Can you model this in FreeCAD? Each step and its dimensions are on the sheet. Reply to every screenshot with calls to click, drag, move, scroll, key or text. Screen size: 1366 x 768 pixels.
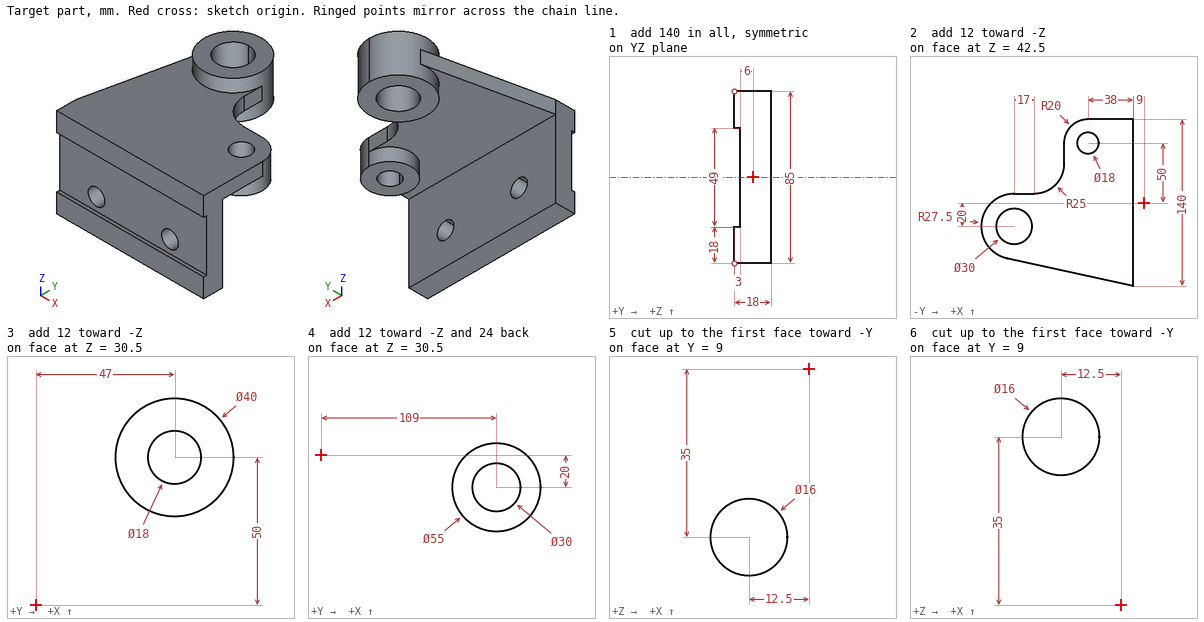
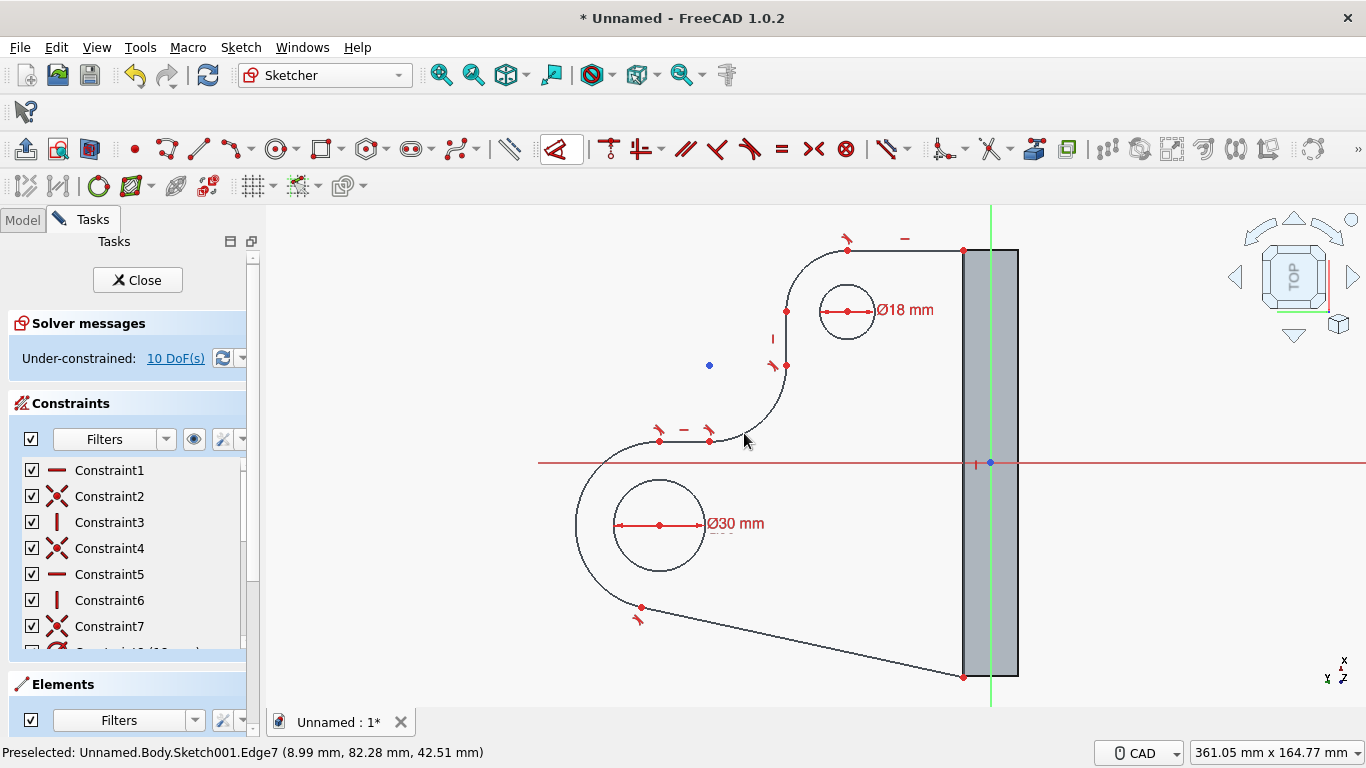
click(786, 349)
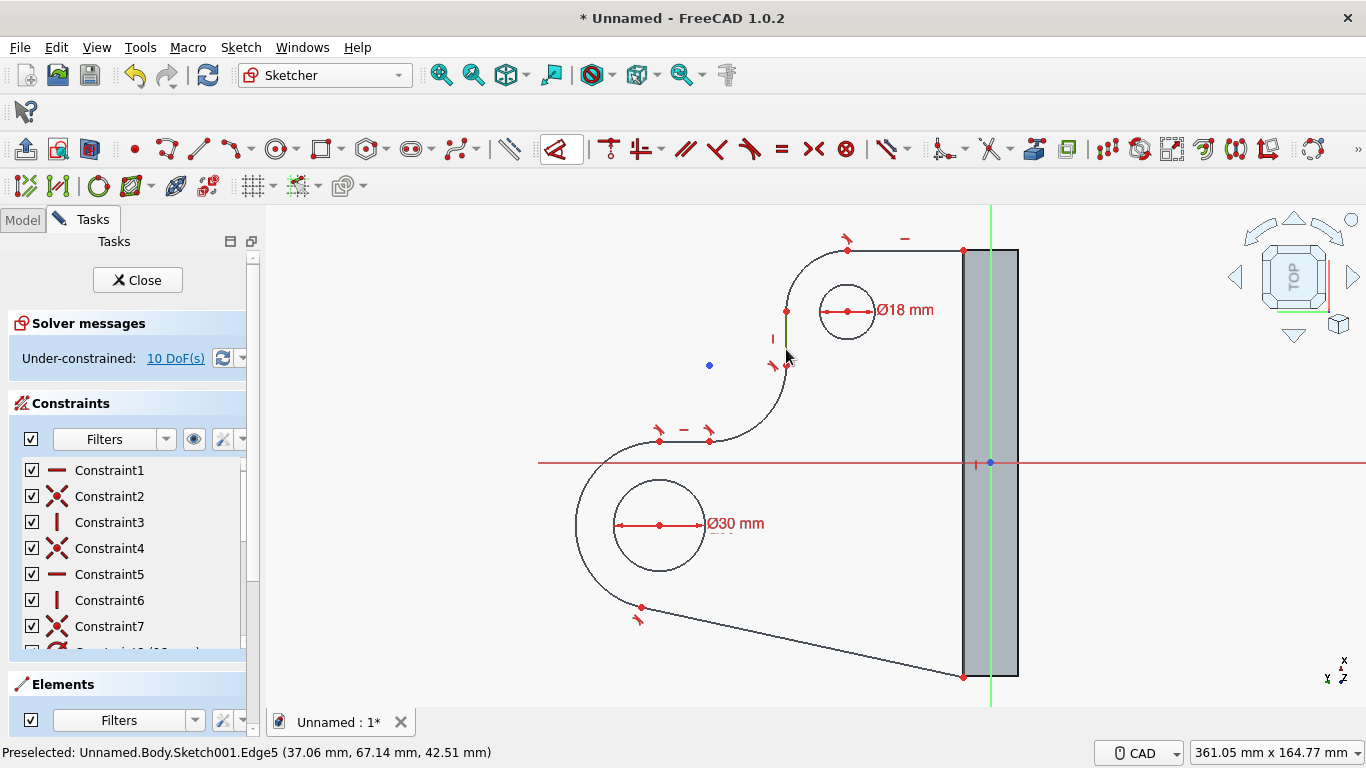
click(820, 257)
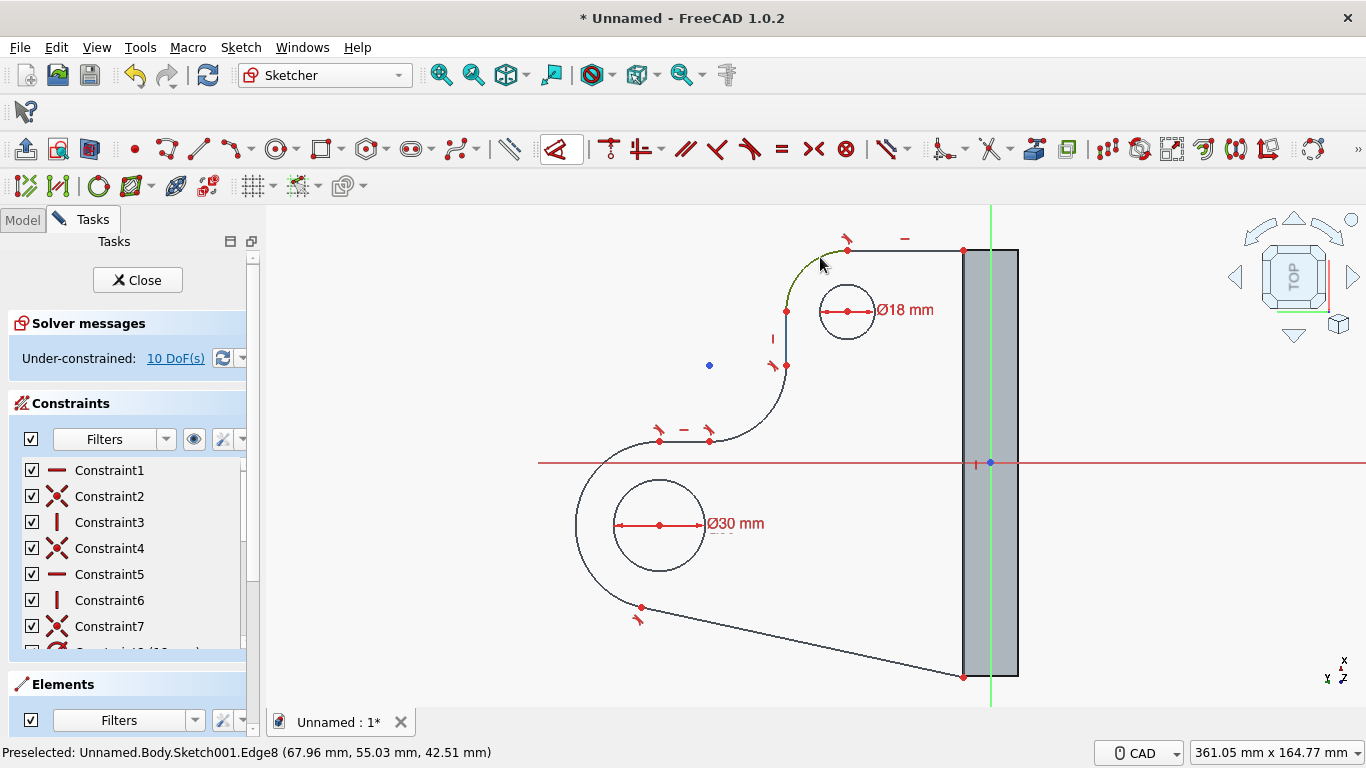
key(t)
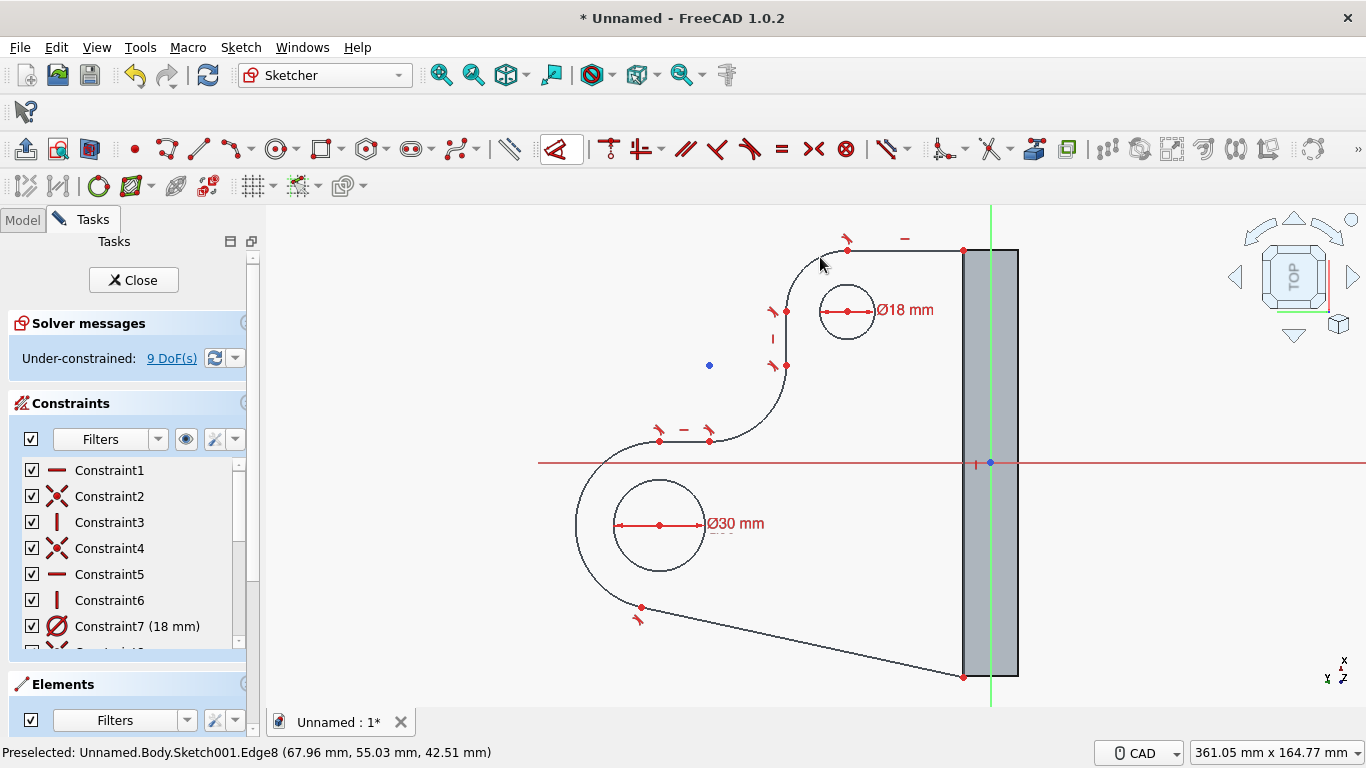
scroll(595, 472, up, 3)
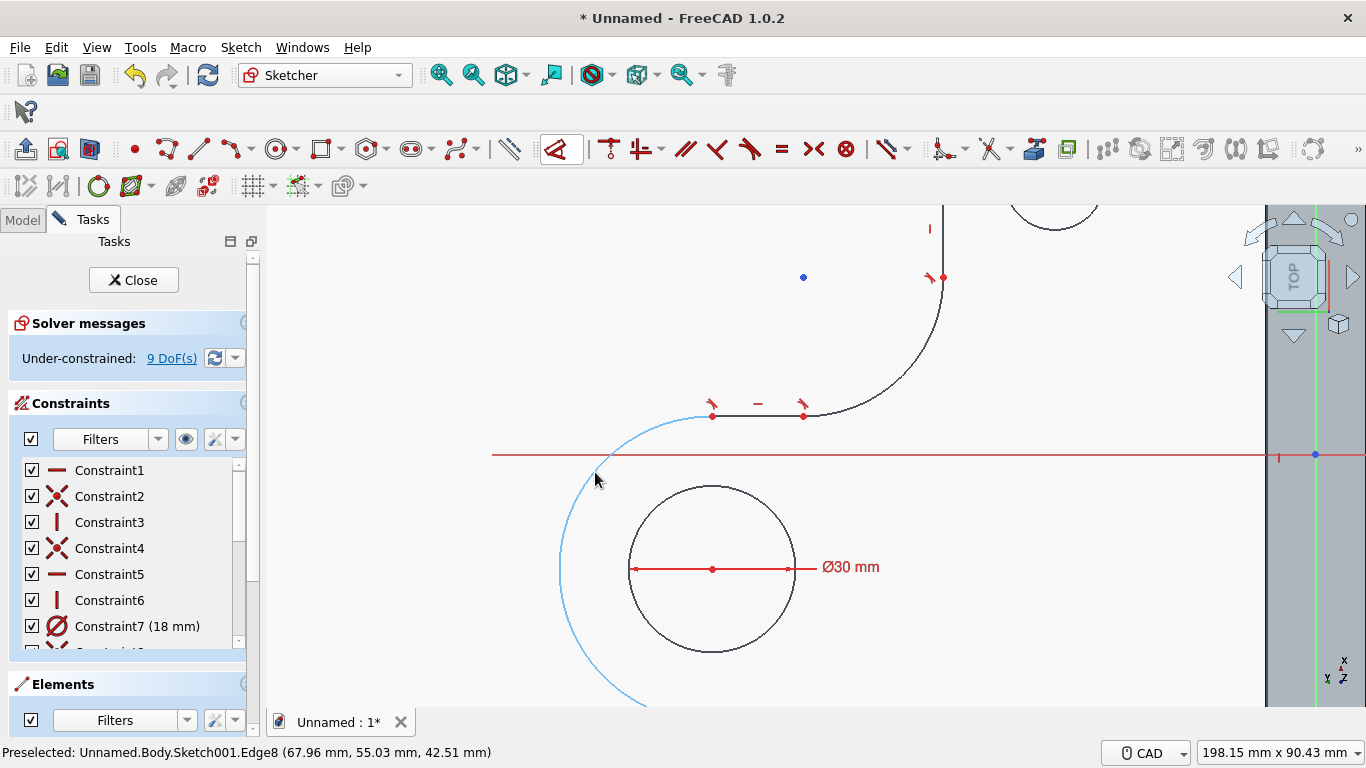
click(595, 472)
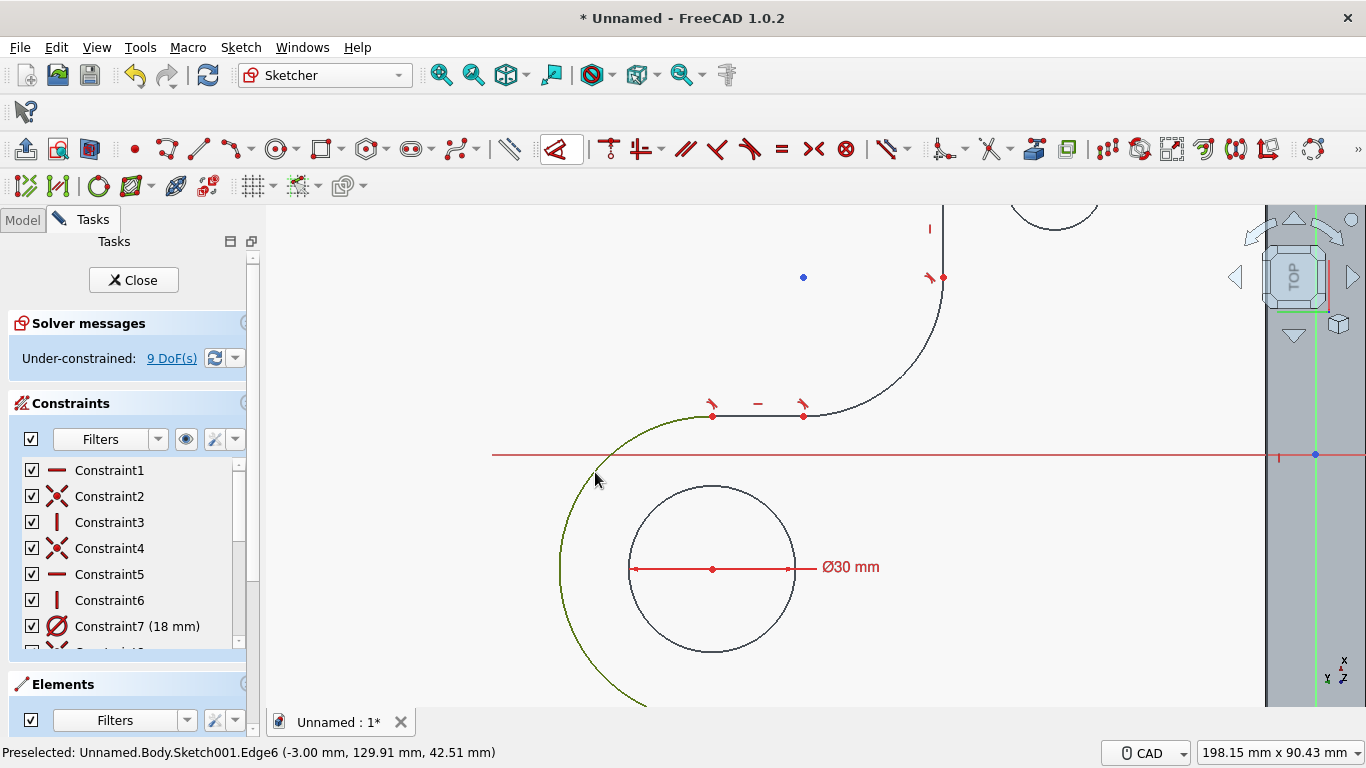
key(k)
key(r)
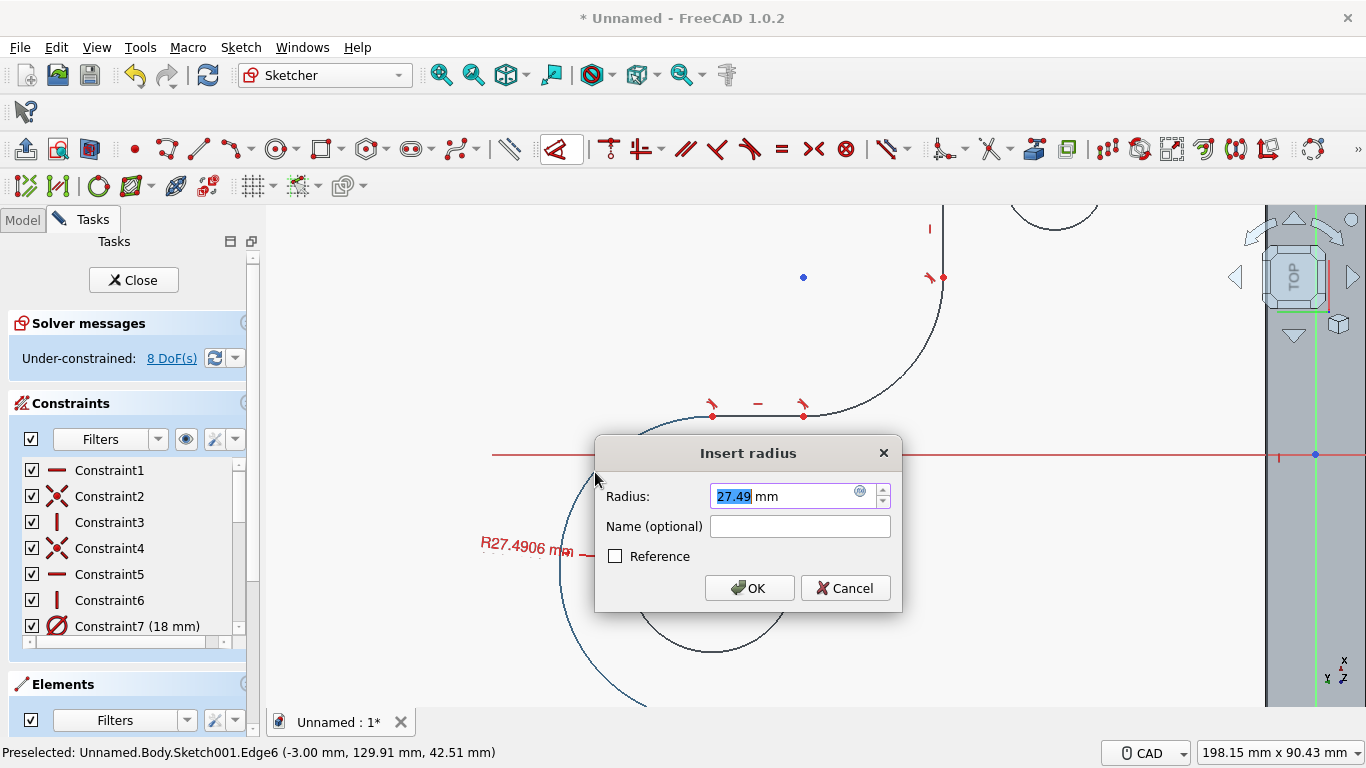
text(27.5)
key(Return)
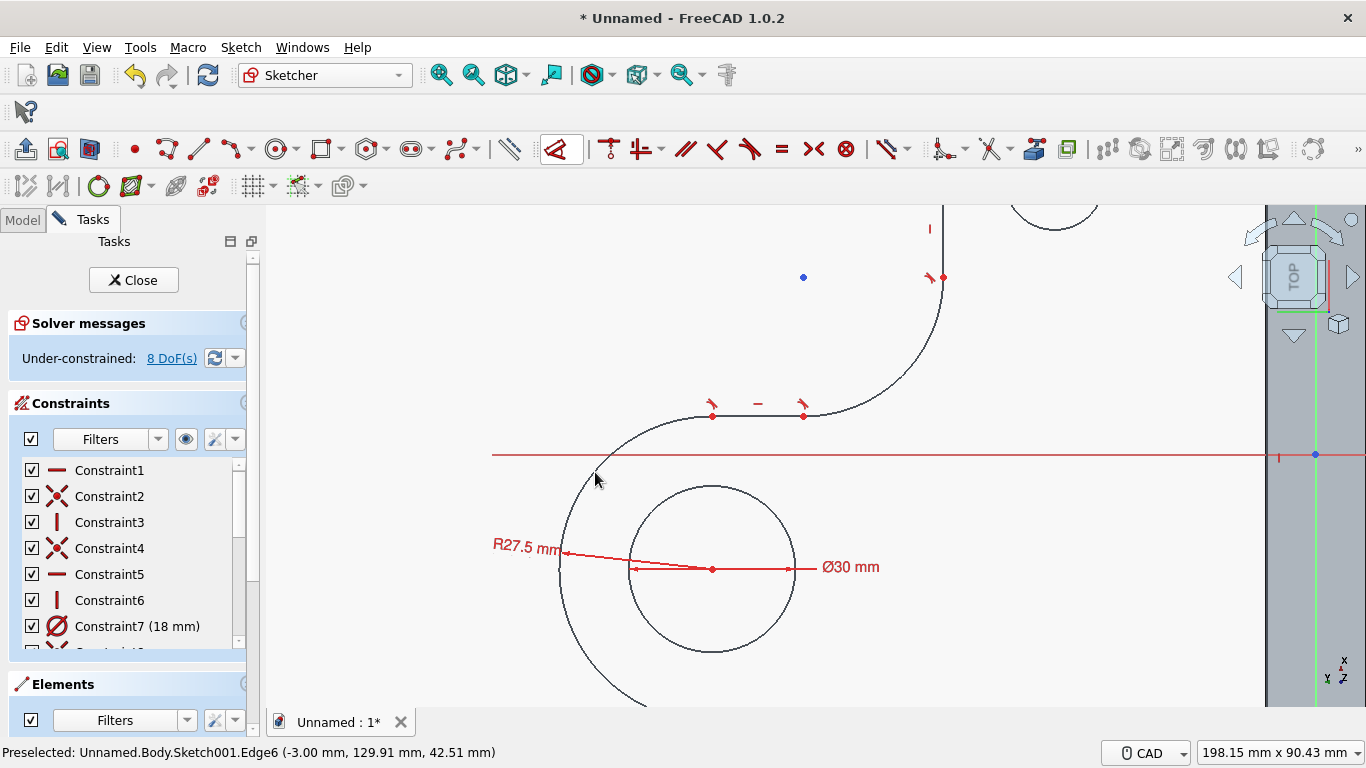
click(867, 401)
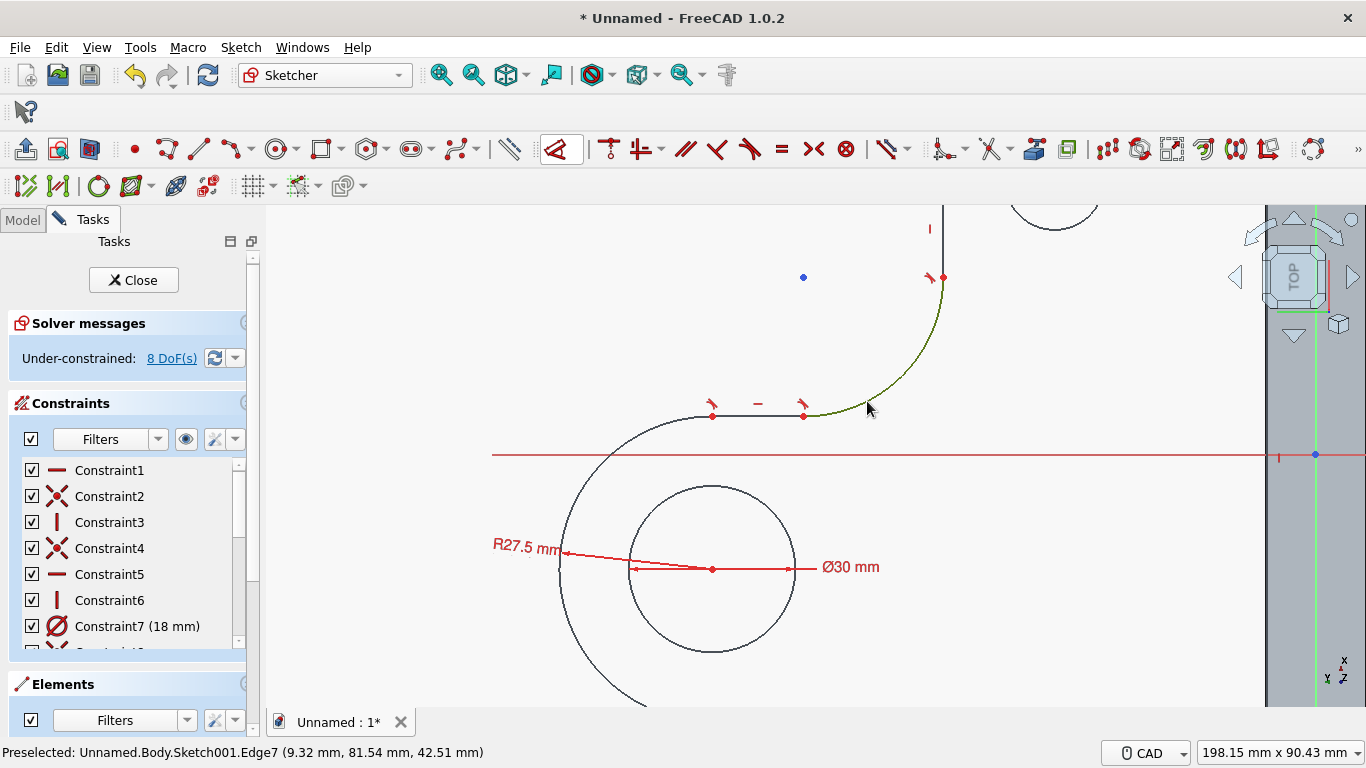
key(k)
key(r)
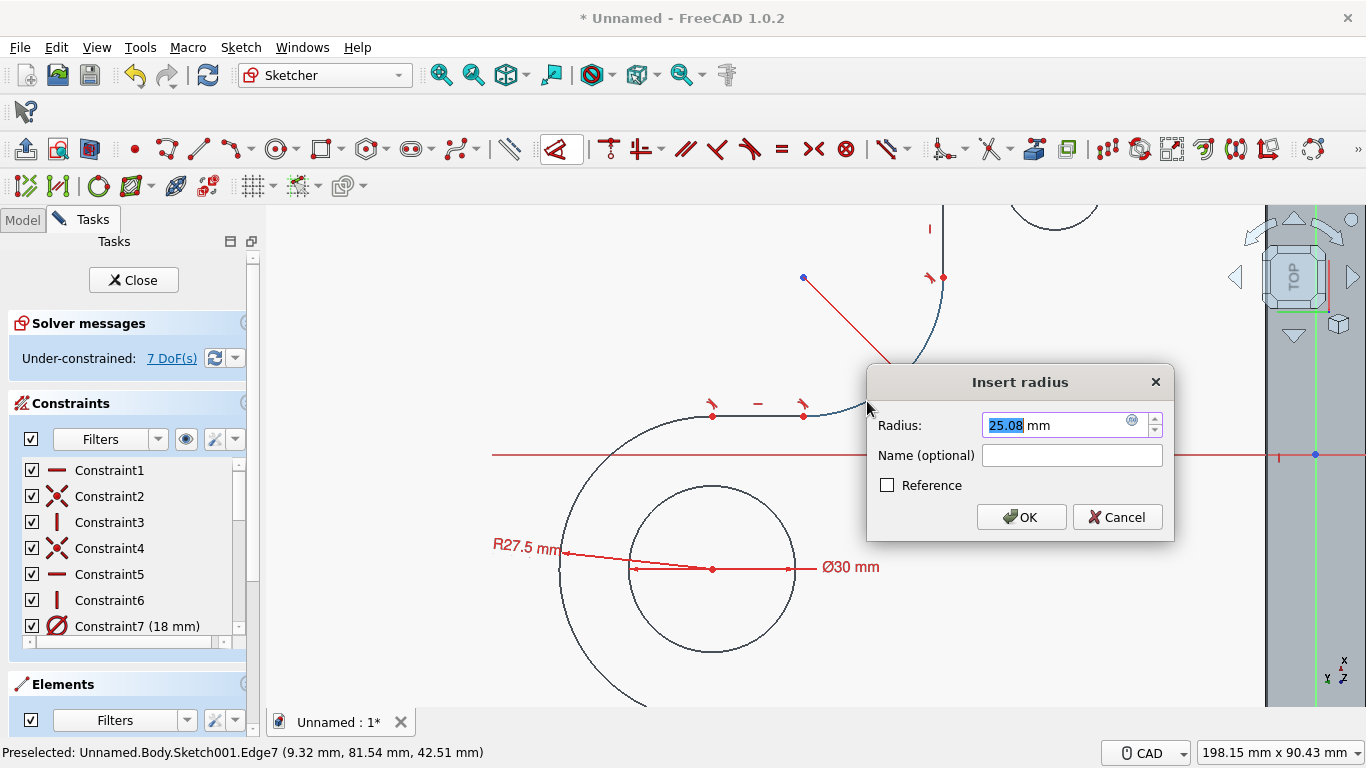
text(25)
key(Return)